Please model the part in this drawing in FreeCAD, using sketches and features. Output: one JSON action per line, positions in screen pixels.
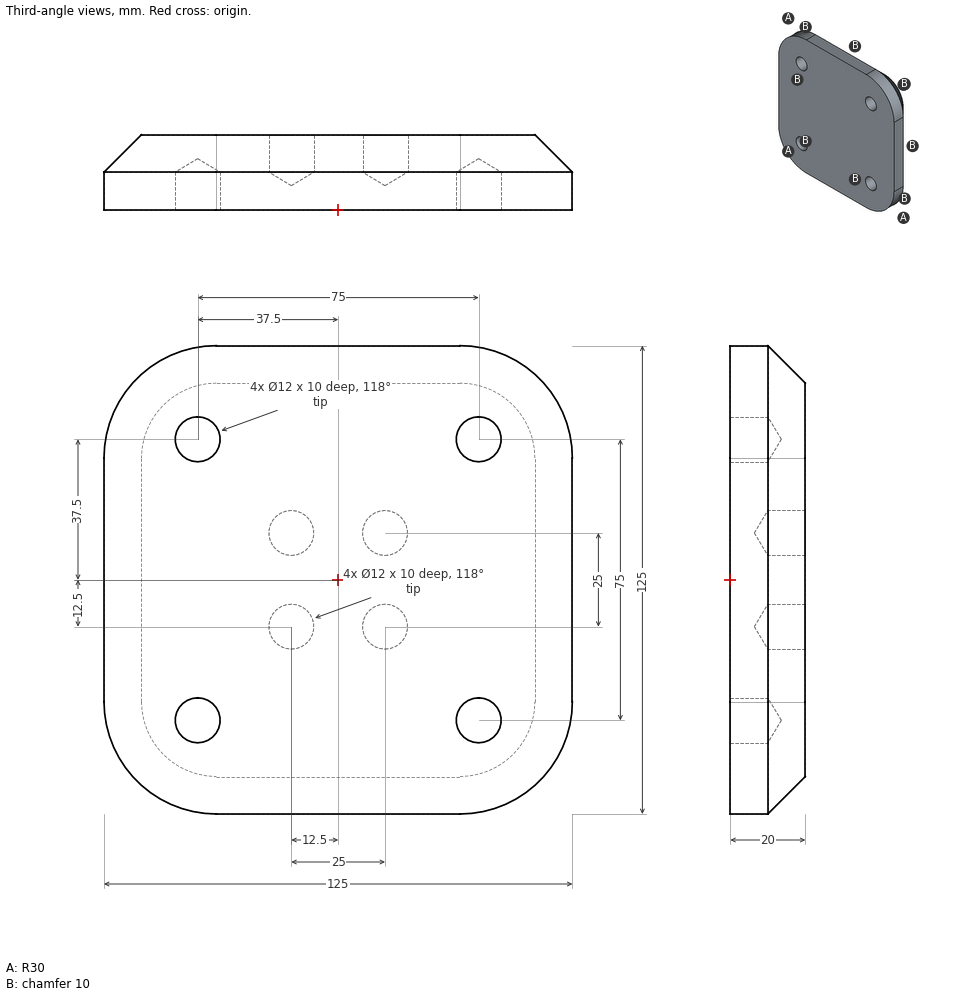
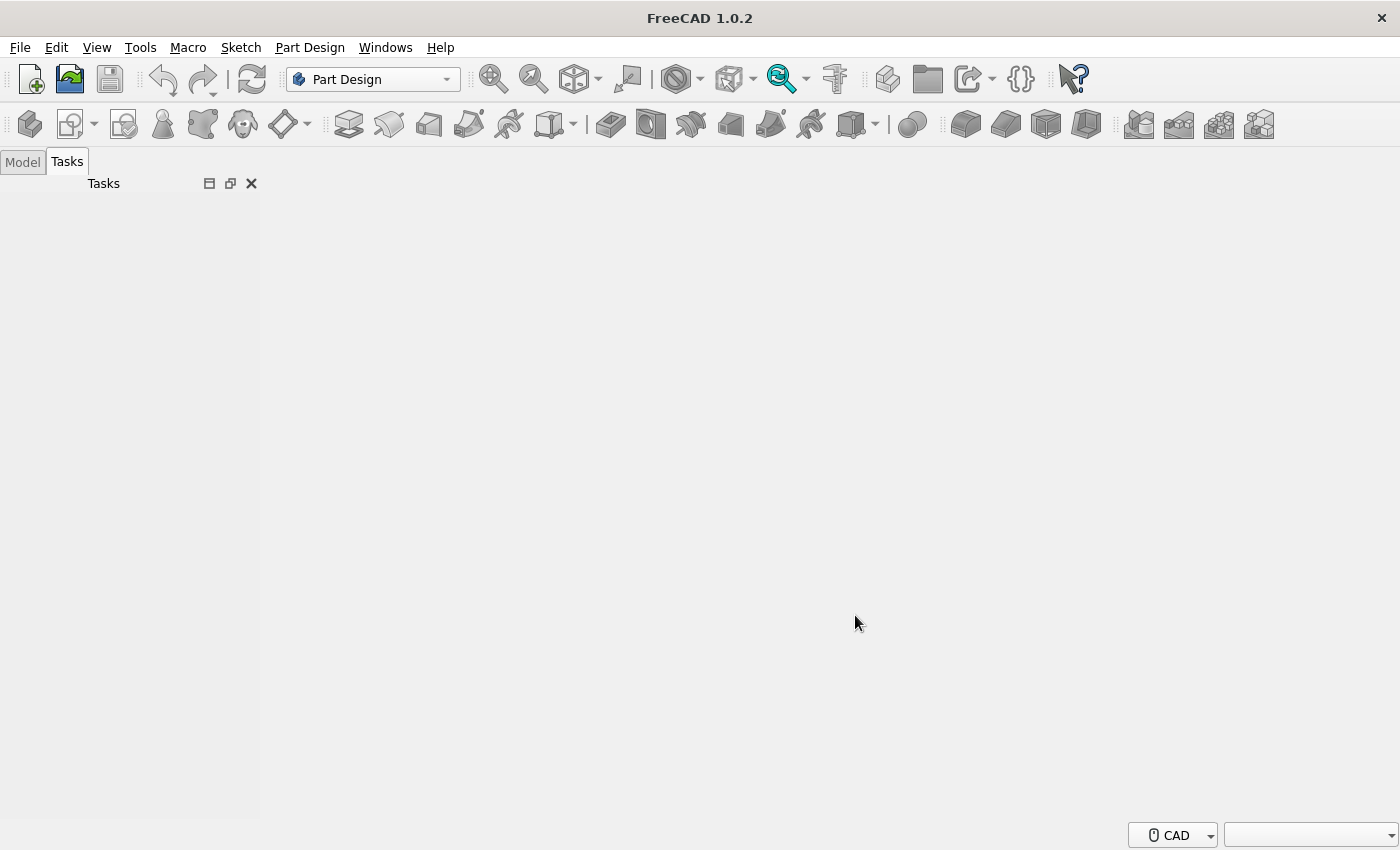
{"action": "left_click", "coordinate": [30, 80]}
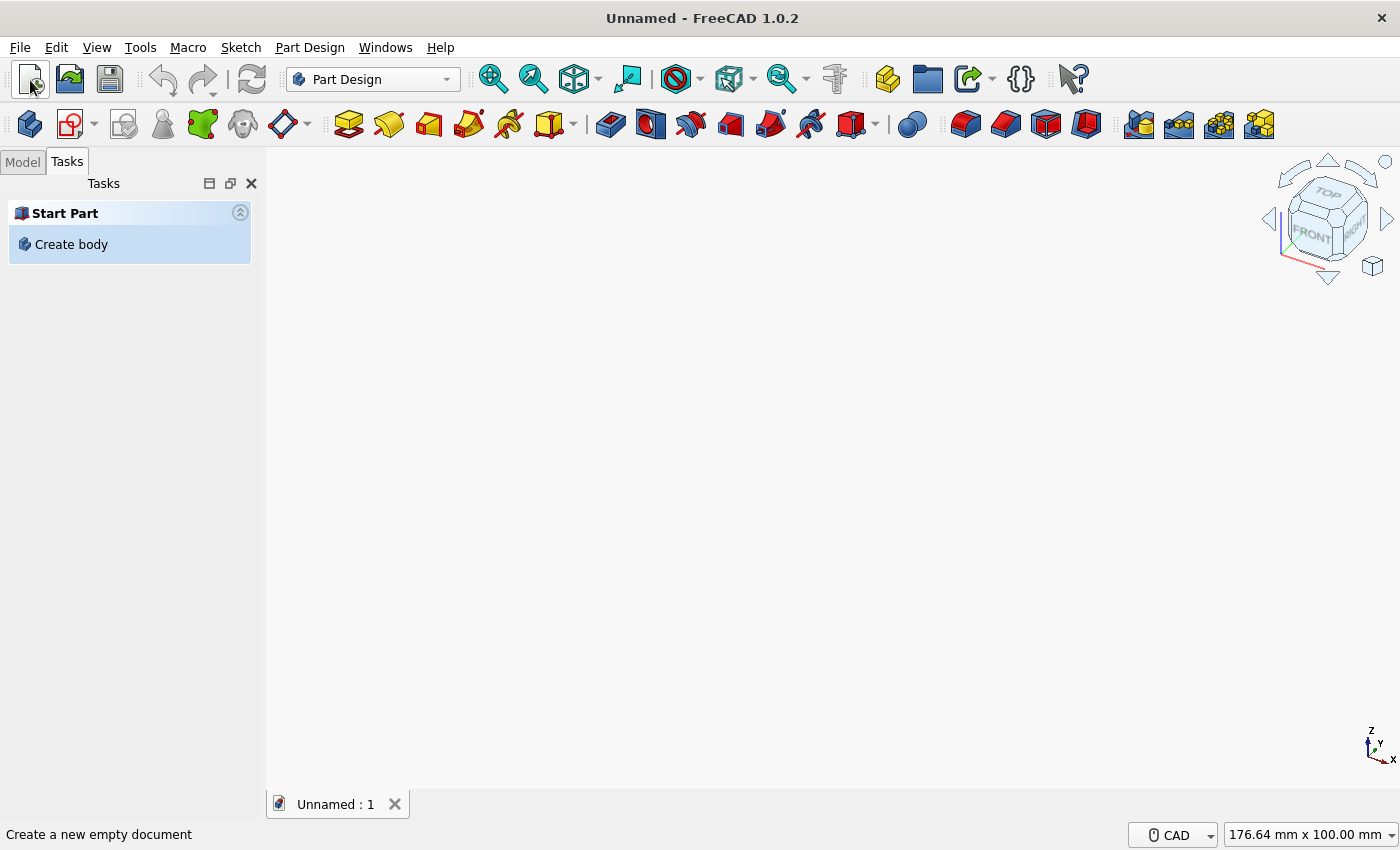
{"action": "left_click", "coordinate": [70, 124]}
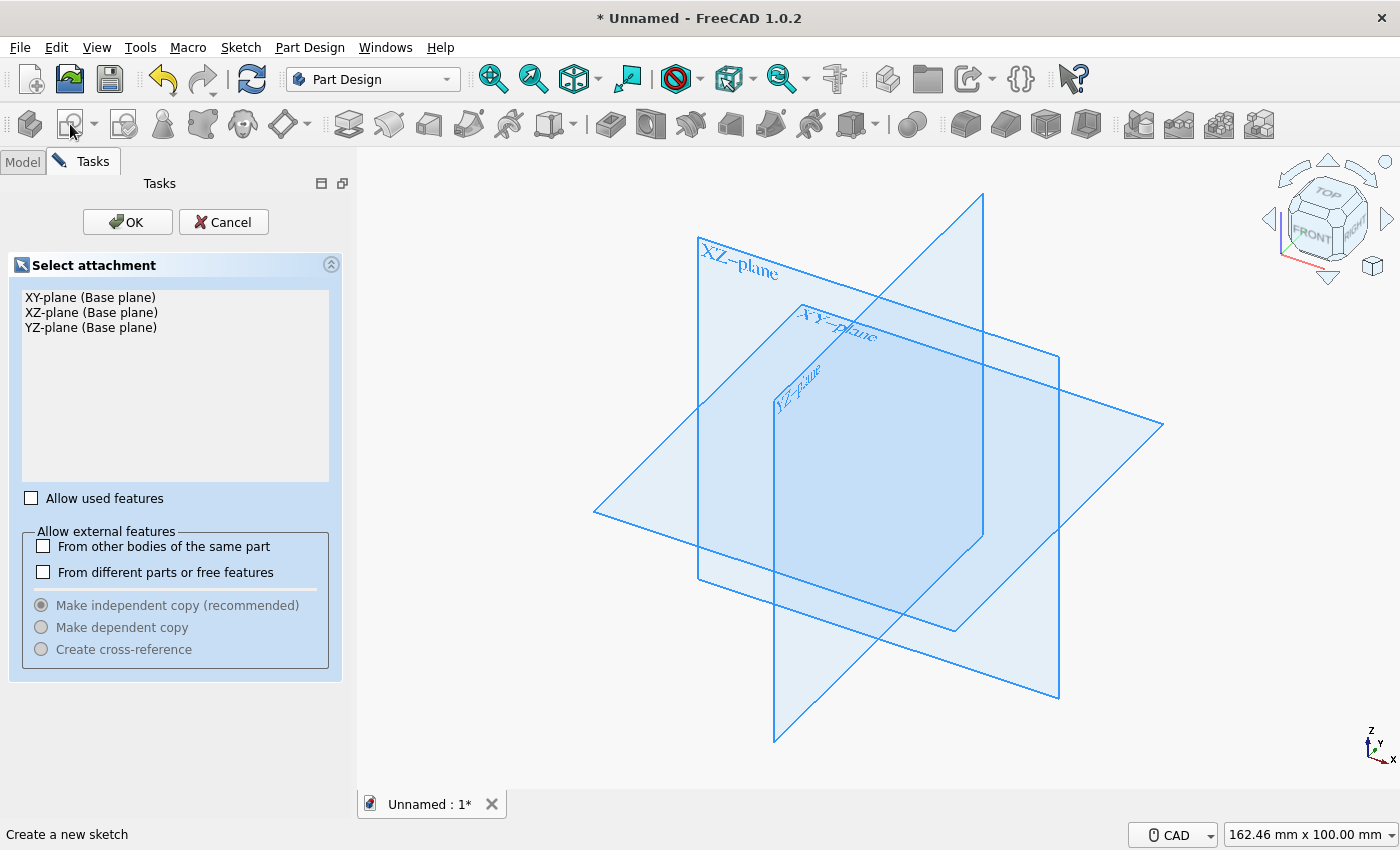
{"action": "left_click", "coordinate": [82, 312]}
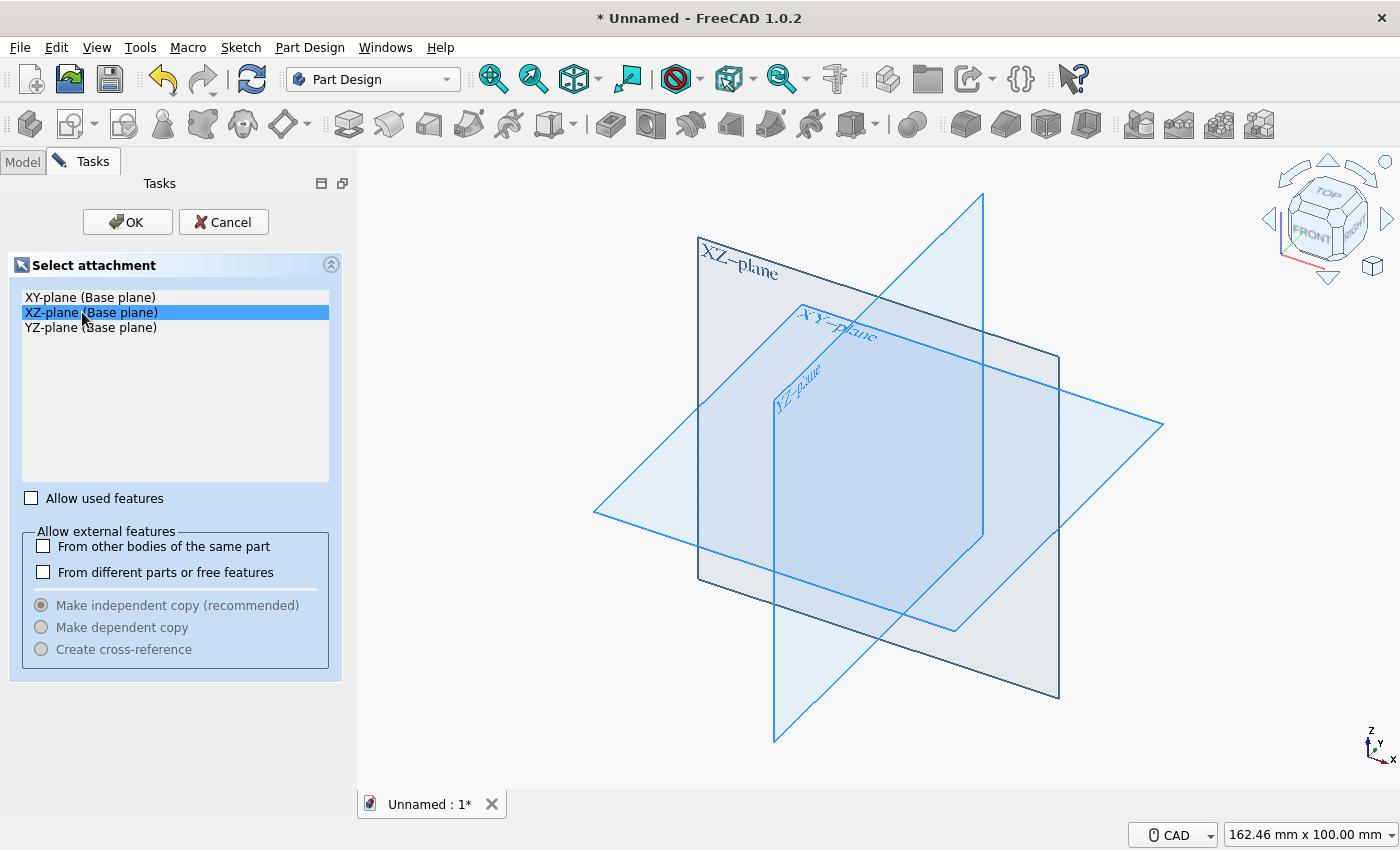
{"action": "left_click", "coordinate": [128, 222]}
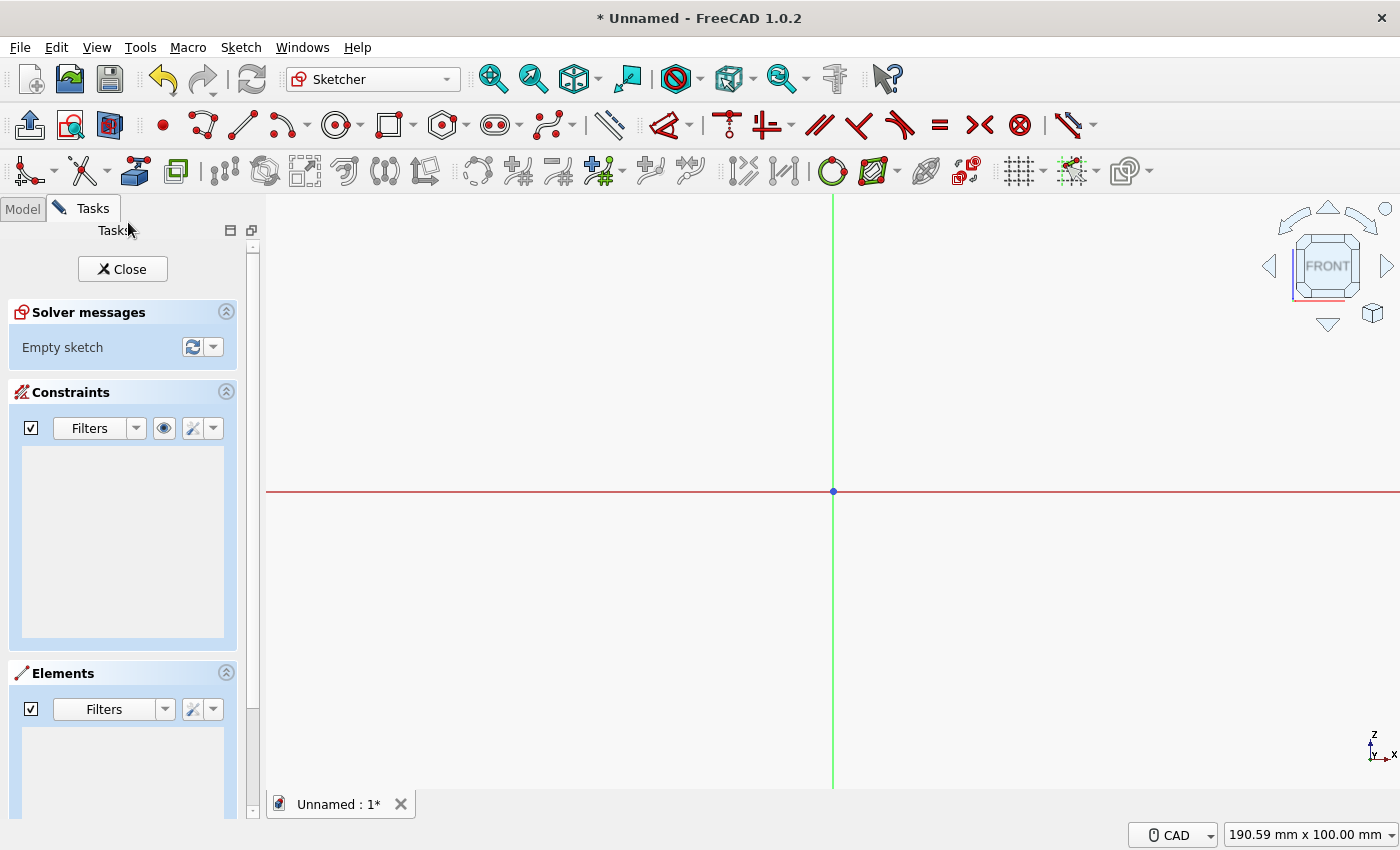
{"action": "scroll", "coordinate": [681, 492], "scroll_direction": "down", "scroll_amount": 3}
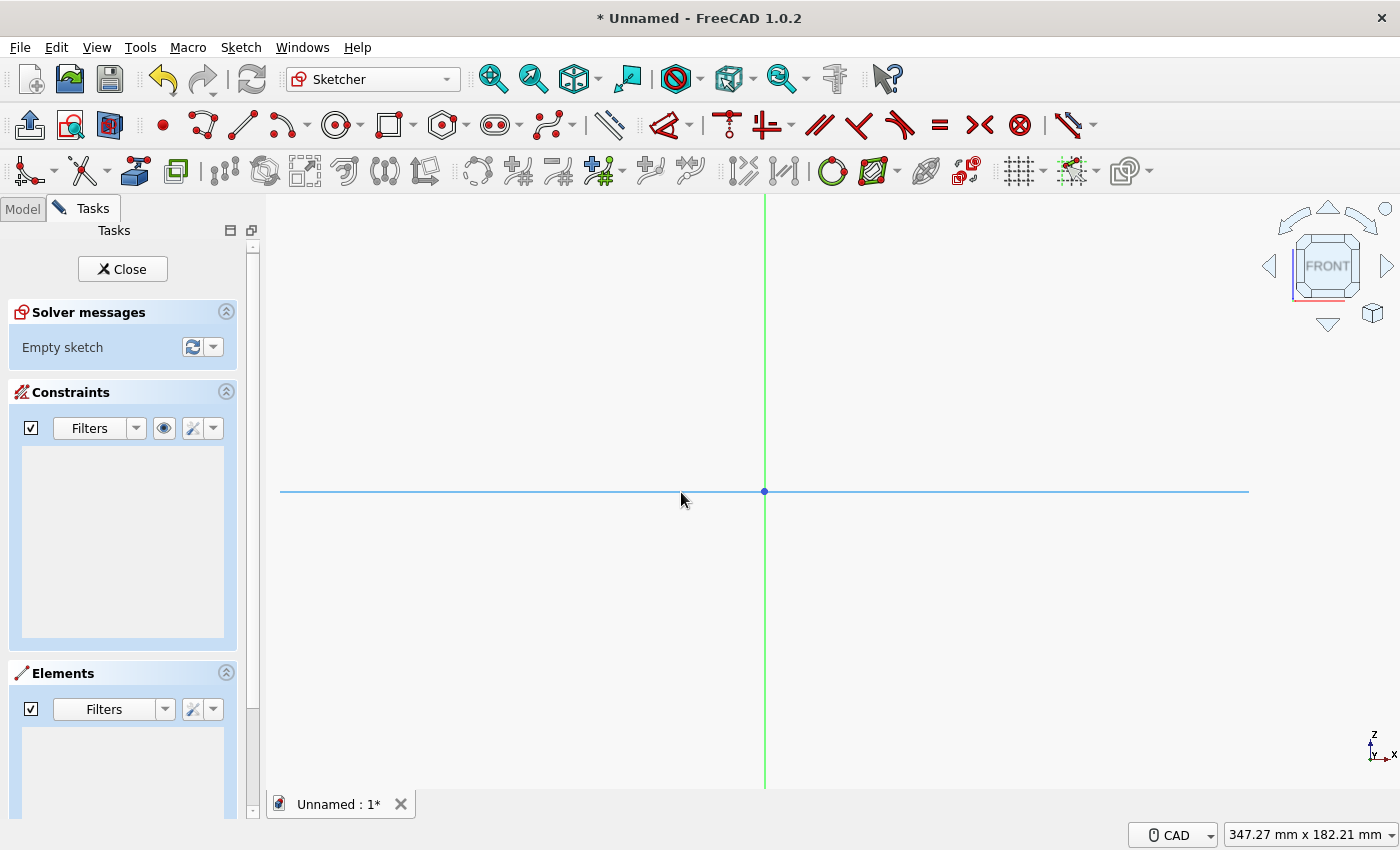
{"action": "left_click", "coordinate": [416, 126]}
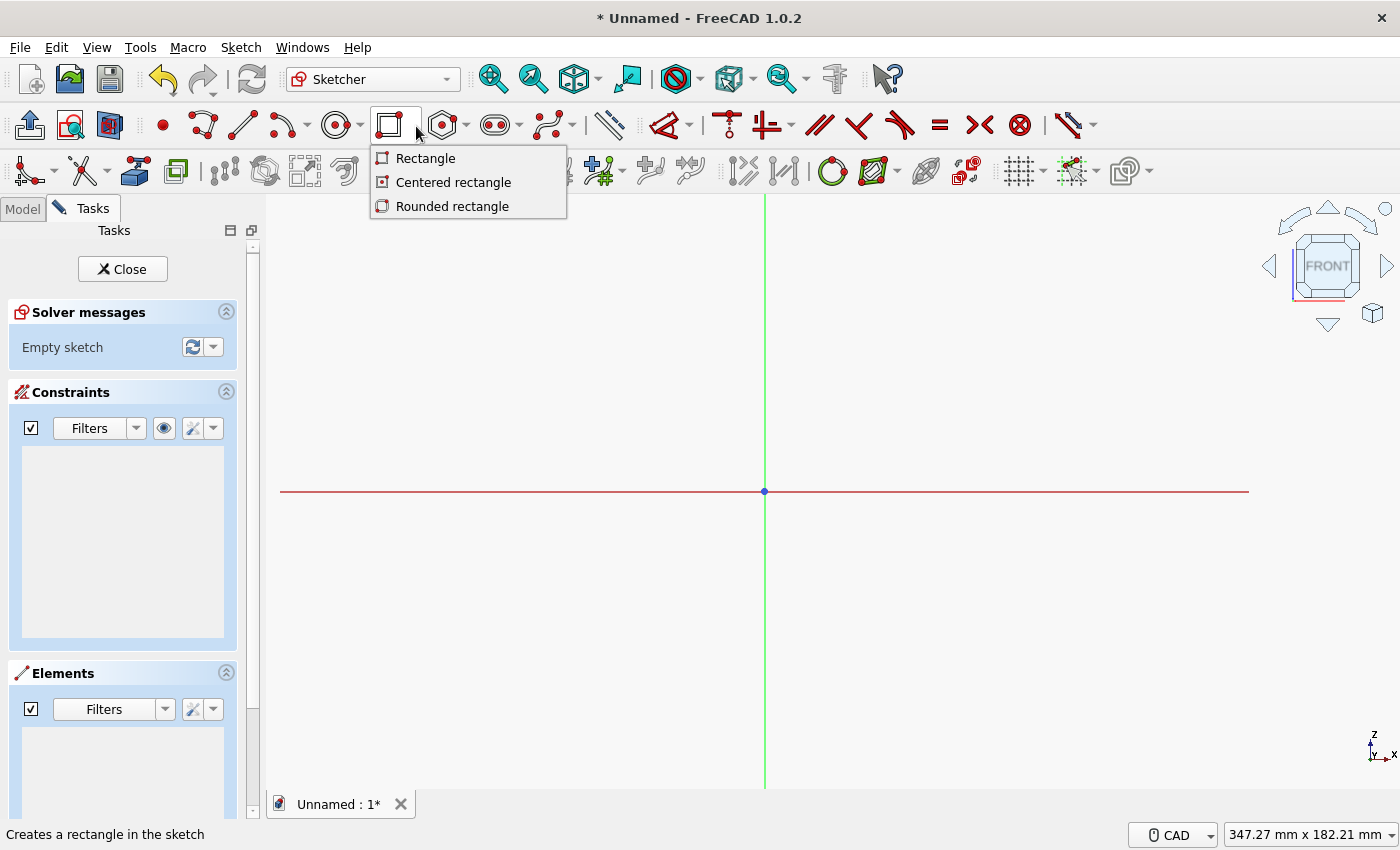
{"action": "left_click", "coordinate": [468, 182]}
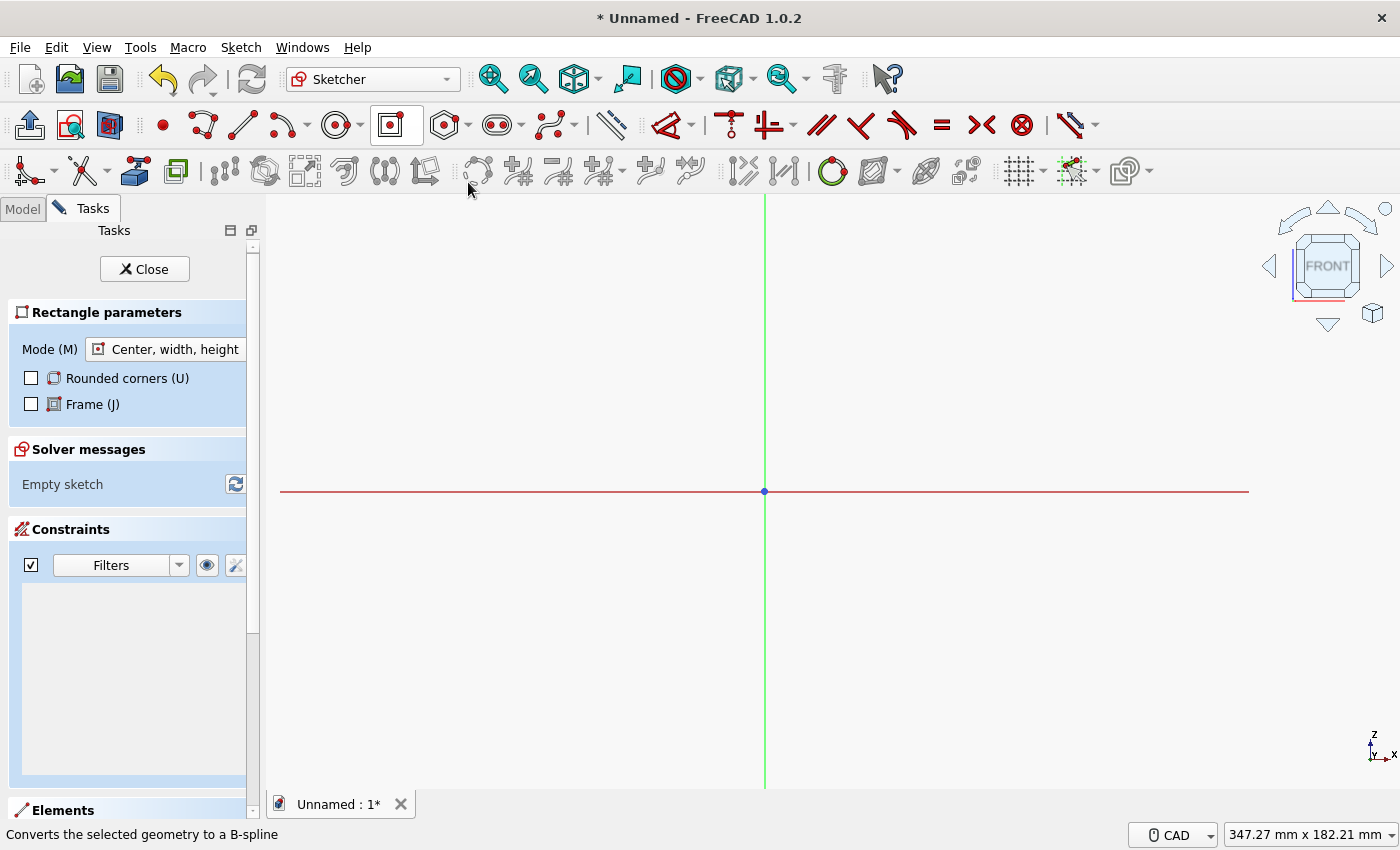
{"action": "left_click", "coordinate": [765, 492]}
{"action": "left_click", "coordinate": [969, 288]}
{"action": "key", "text": "Escape"}